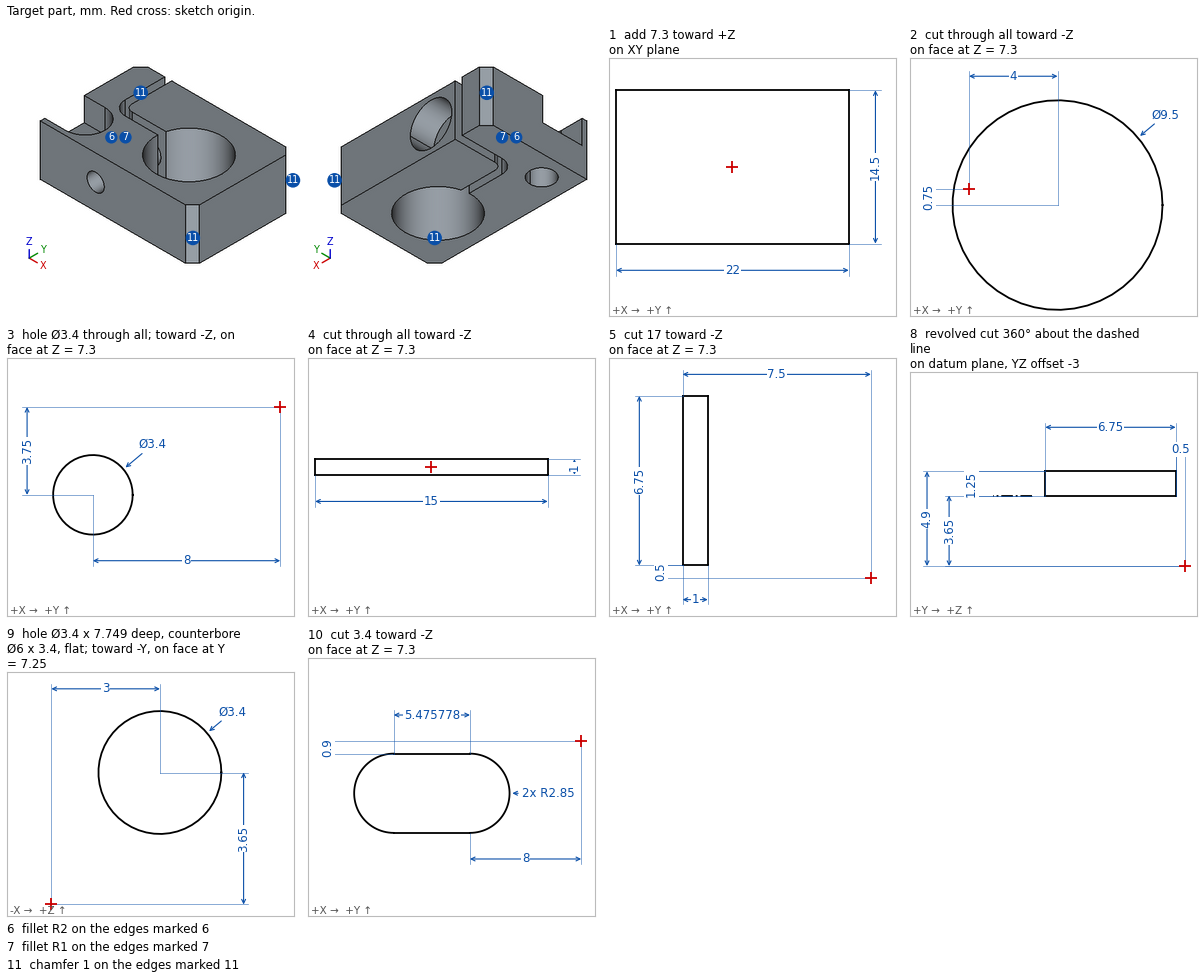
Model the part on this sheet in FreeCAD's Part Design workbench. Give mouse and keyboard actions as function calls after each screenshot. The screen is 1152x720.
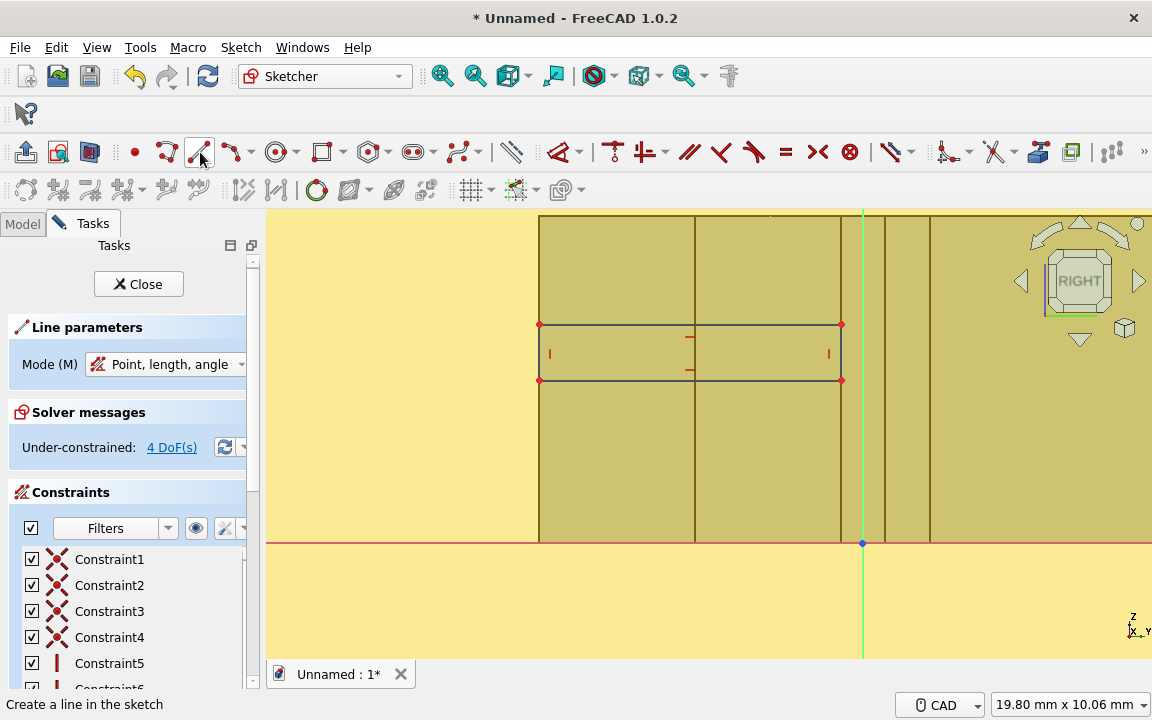
click(508, 380)
click(418, 380)
key(Escape)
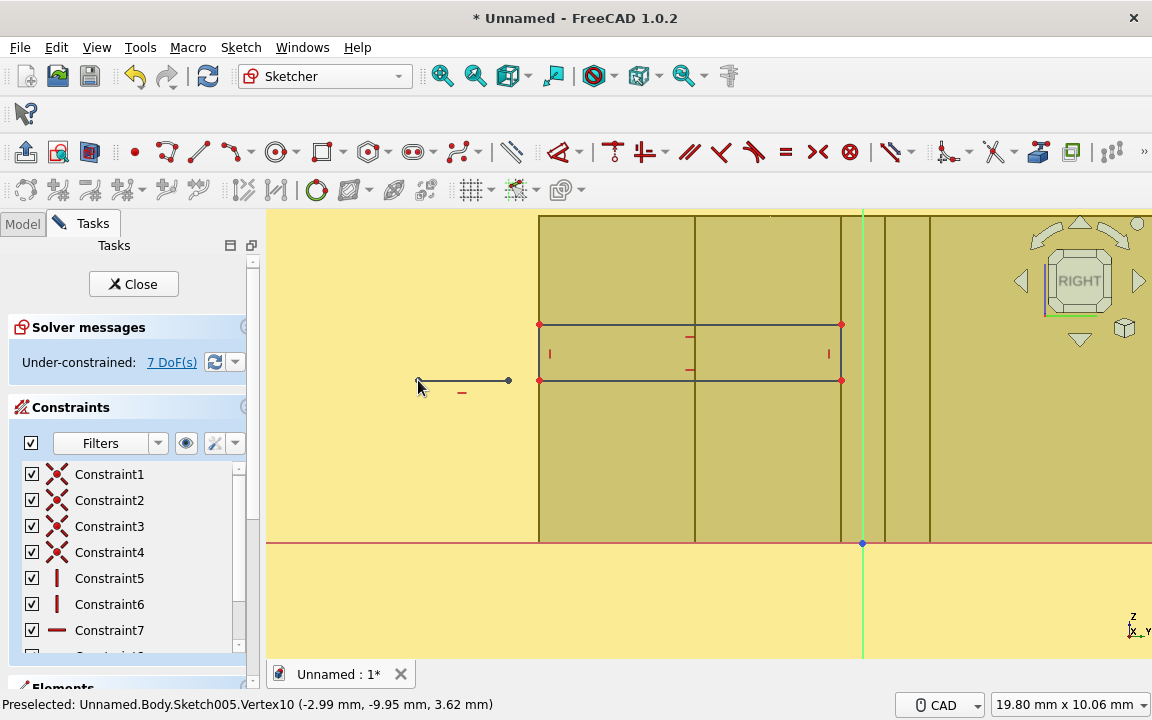
click(481, 381)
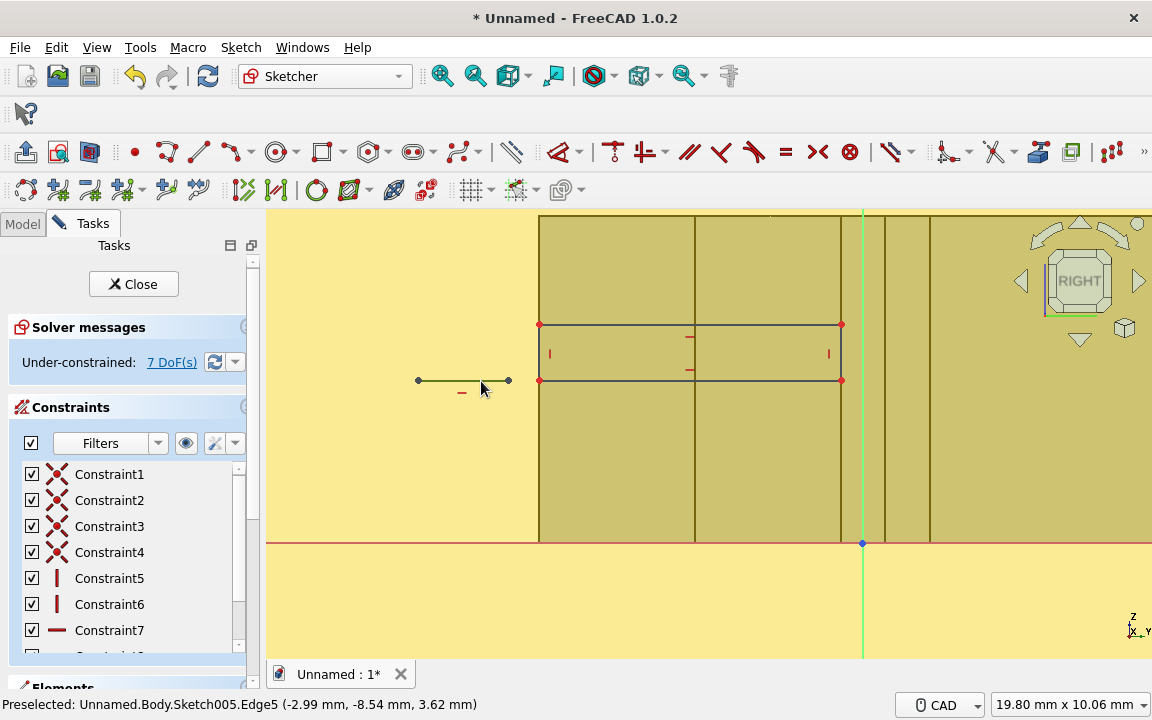
click(512, 152)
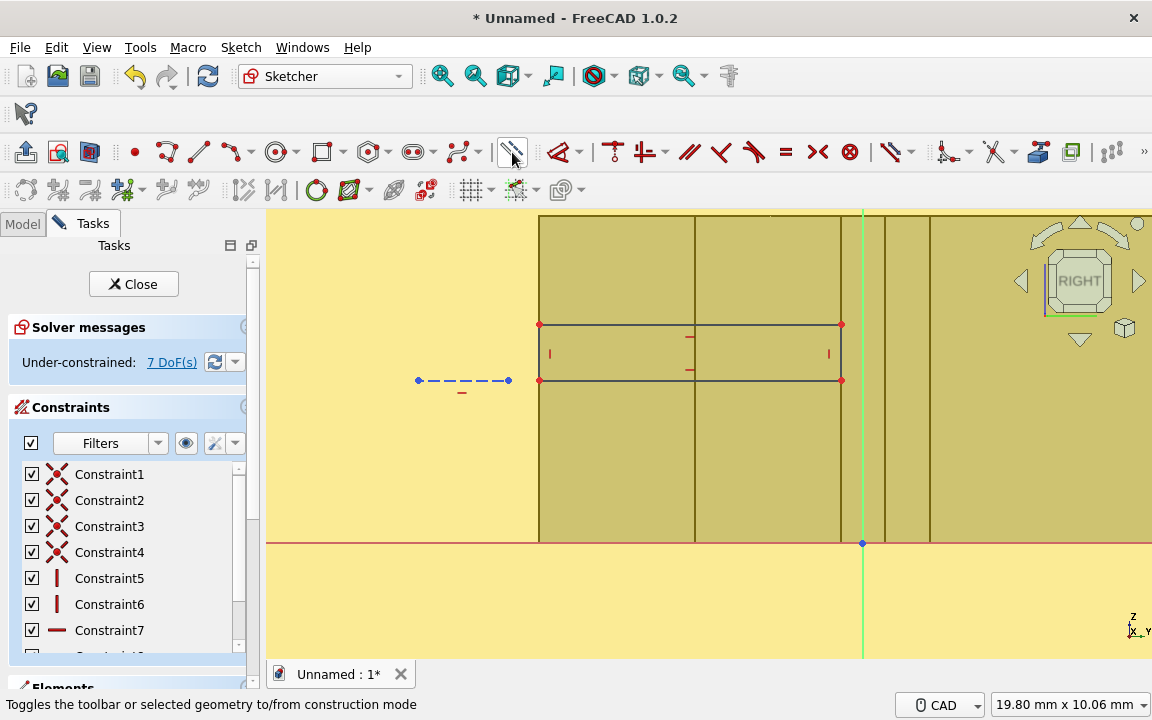
key(d)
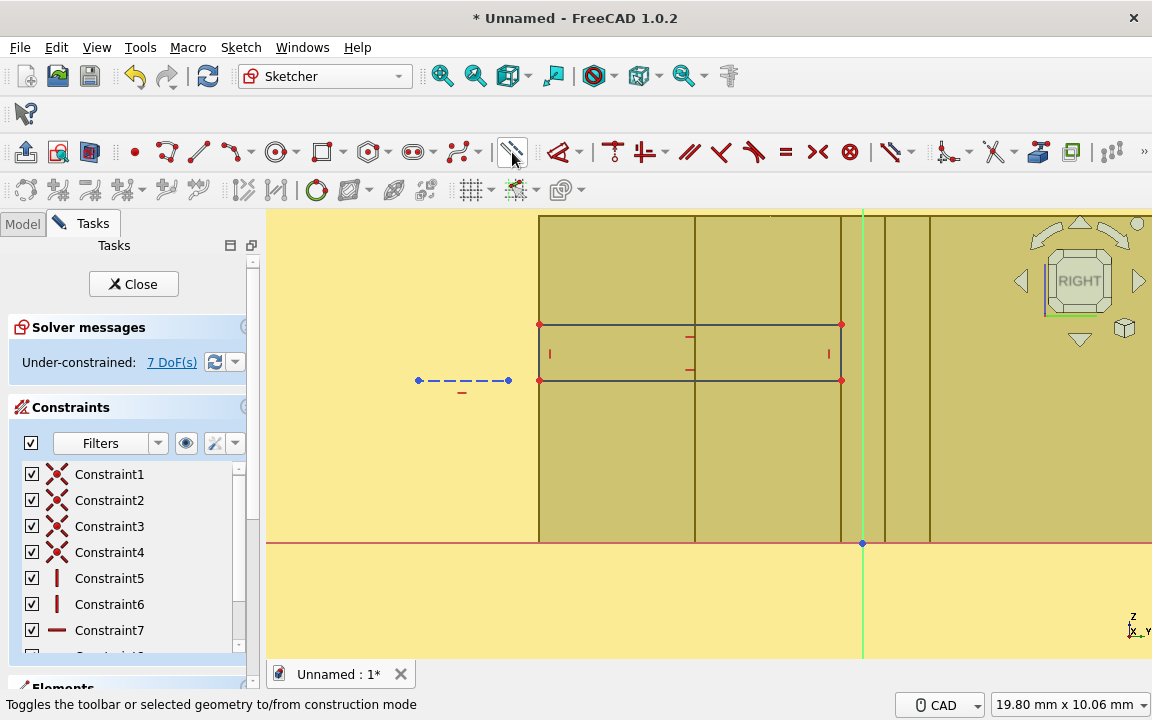
click(539, 342)
click(505, 353)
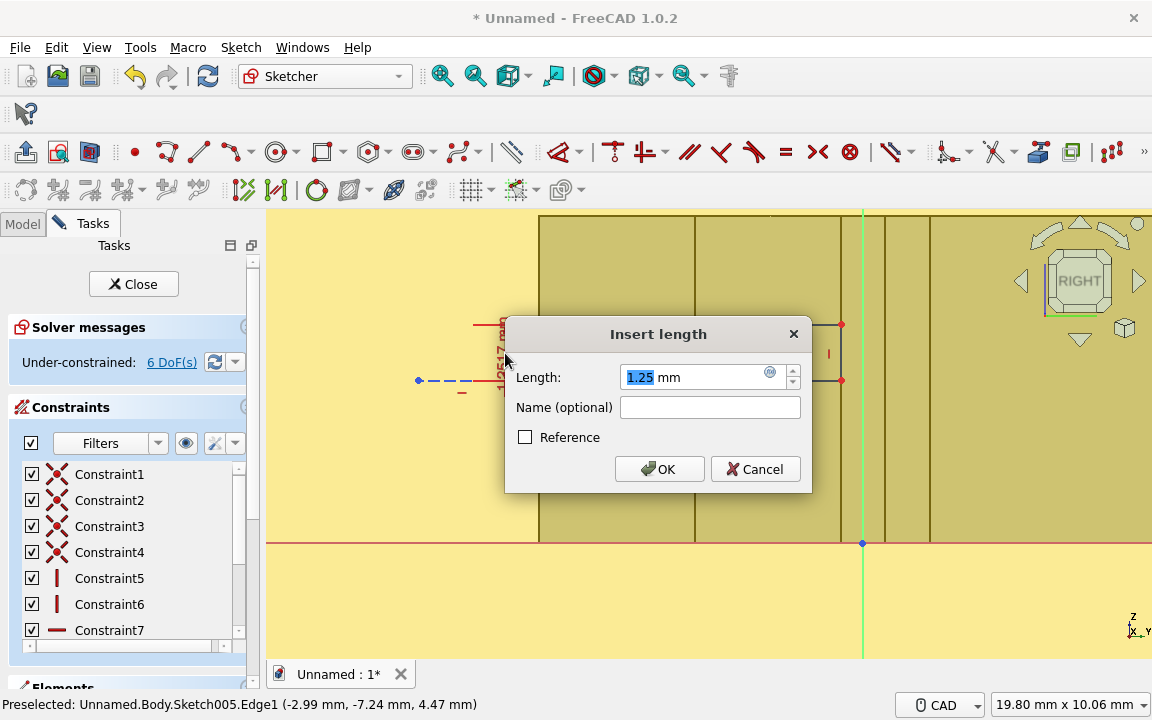
text(1.25)
key(Return)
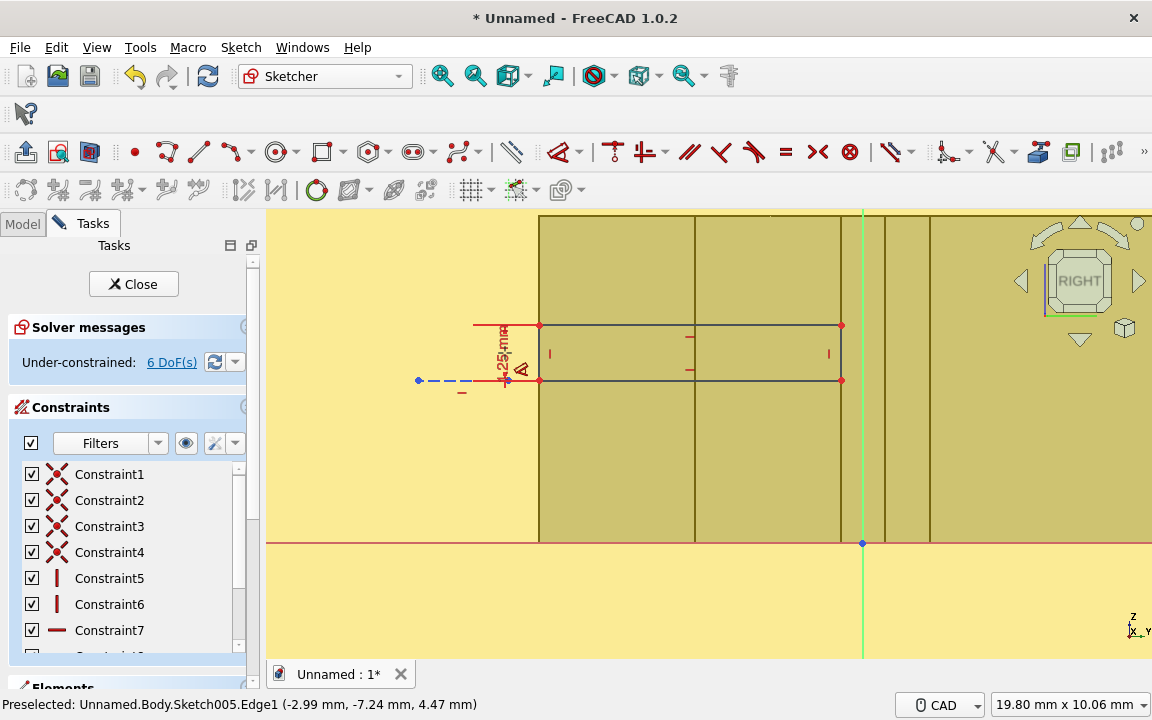
click(630, 381)
click(690, 347)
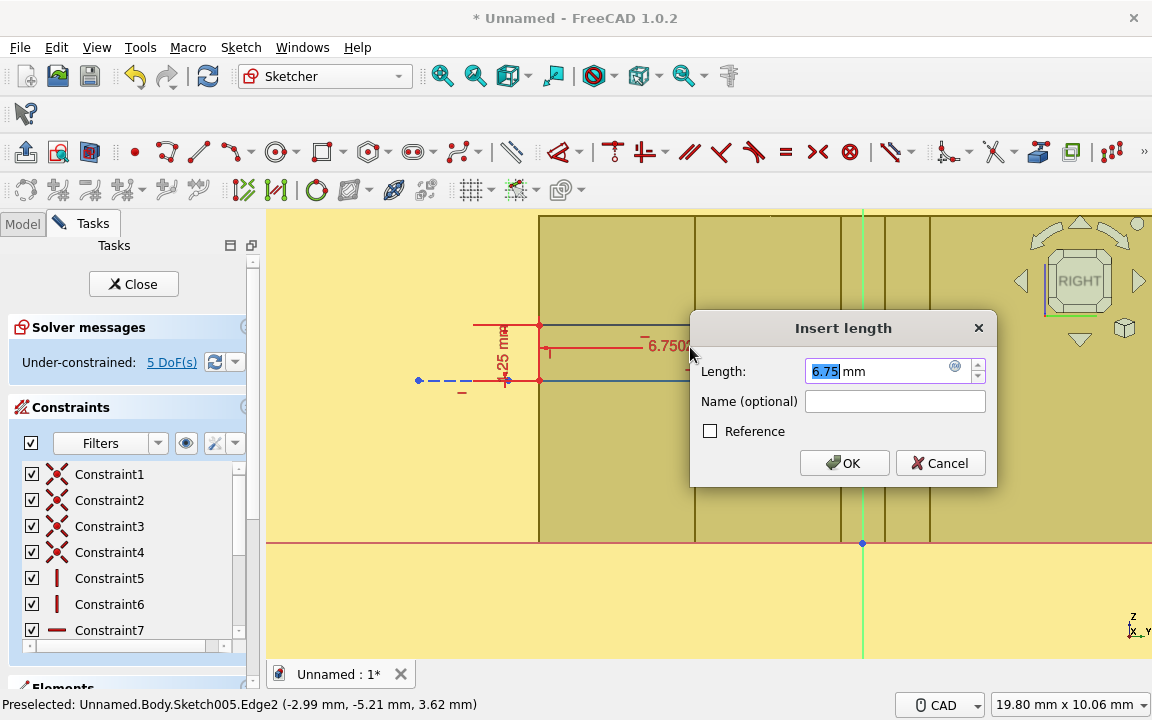
text(6.75)
key(Return)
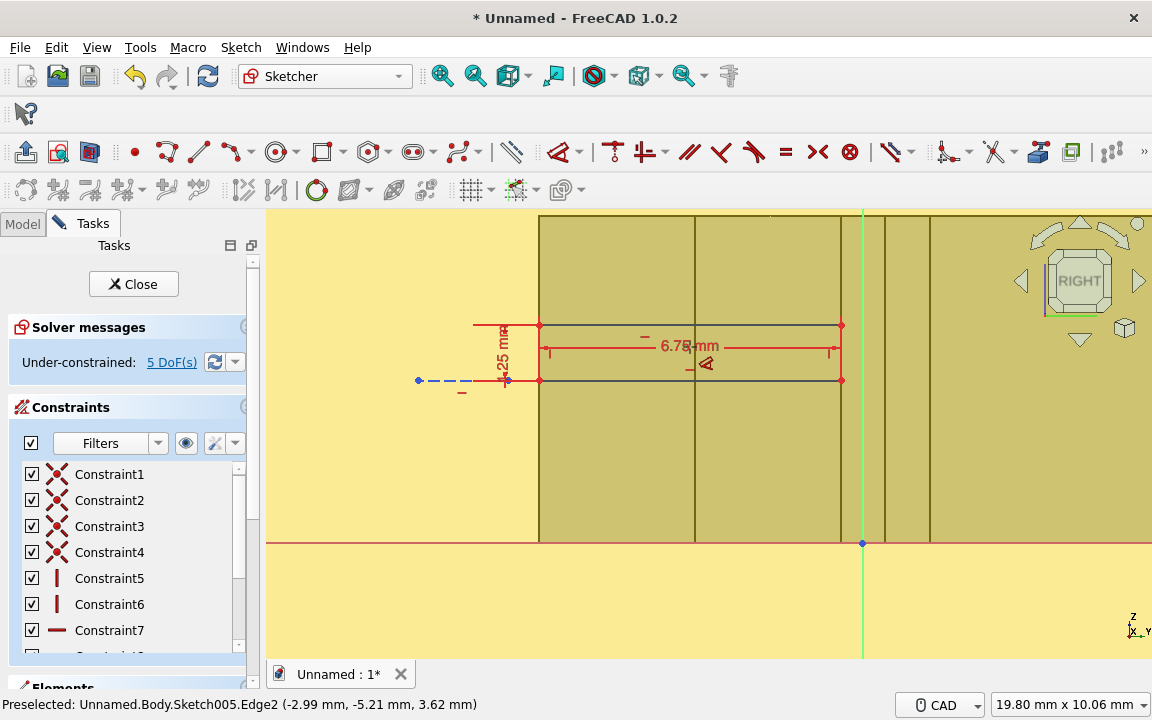
click(539, 325)
click(897, 434)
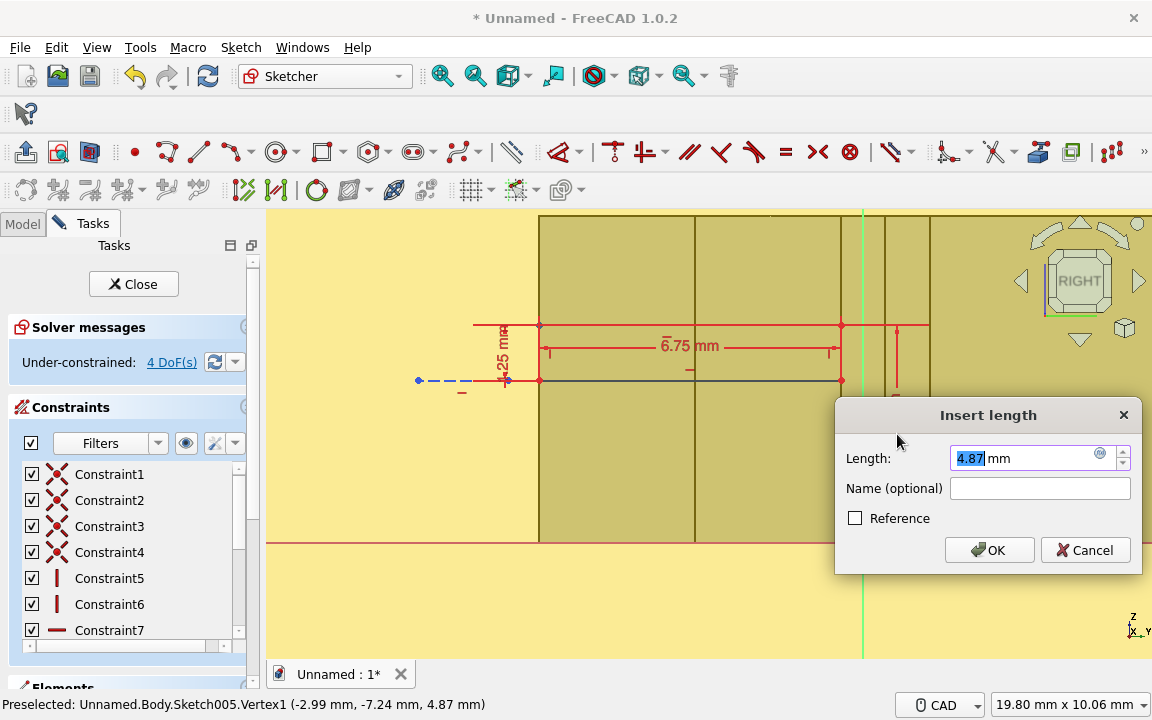
text(4.9)
key(Return)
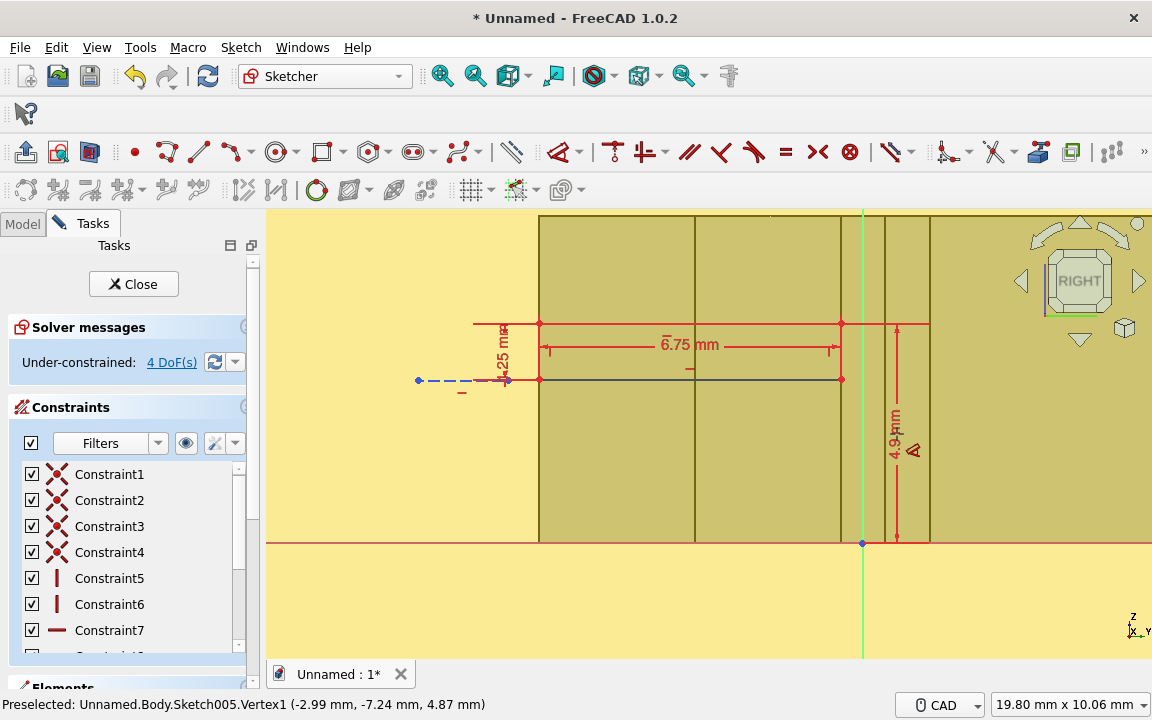
scroll(841, 380, up, 3)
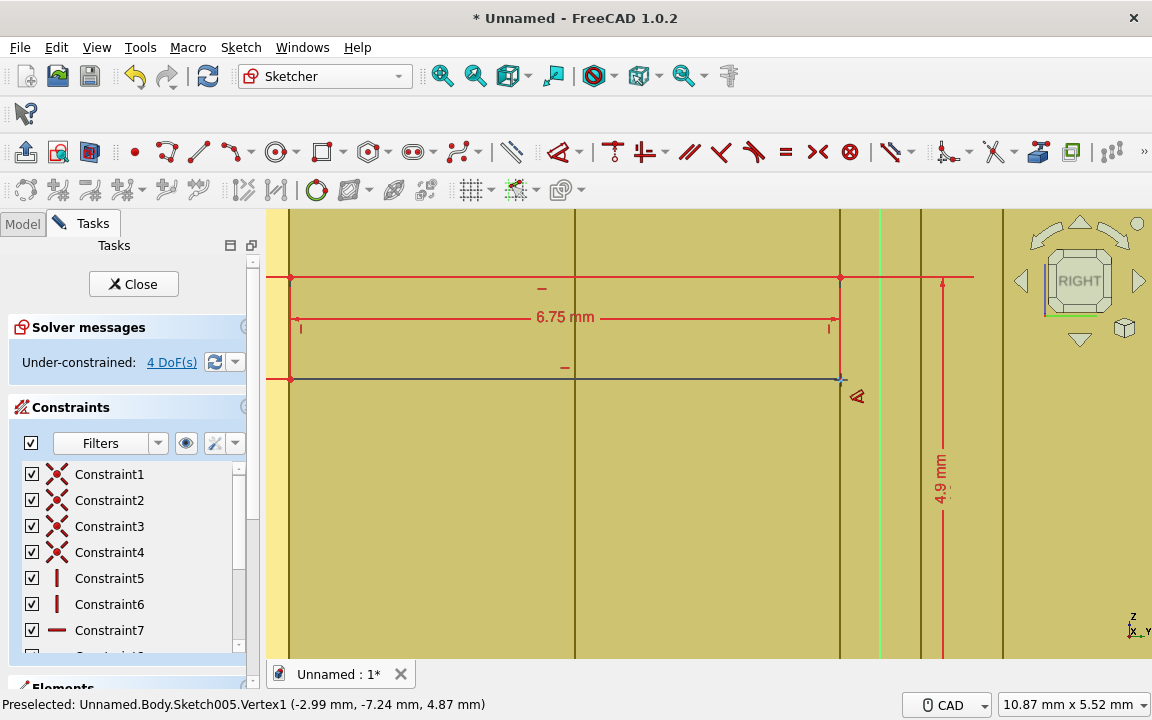
click(840, 379)
click(860, 345)